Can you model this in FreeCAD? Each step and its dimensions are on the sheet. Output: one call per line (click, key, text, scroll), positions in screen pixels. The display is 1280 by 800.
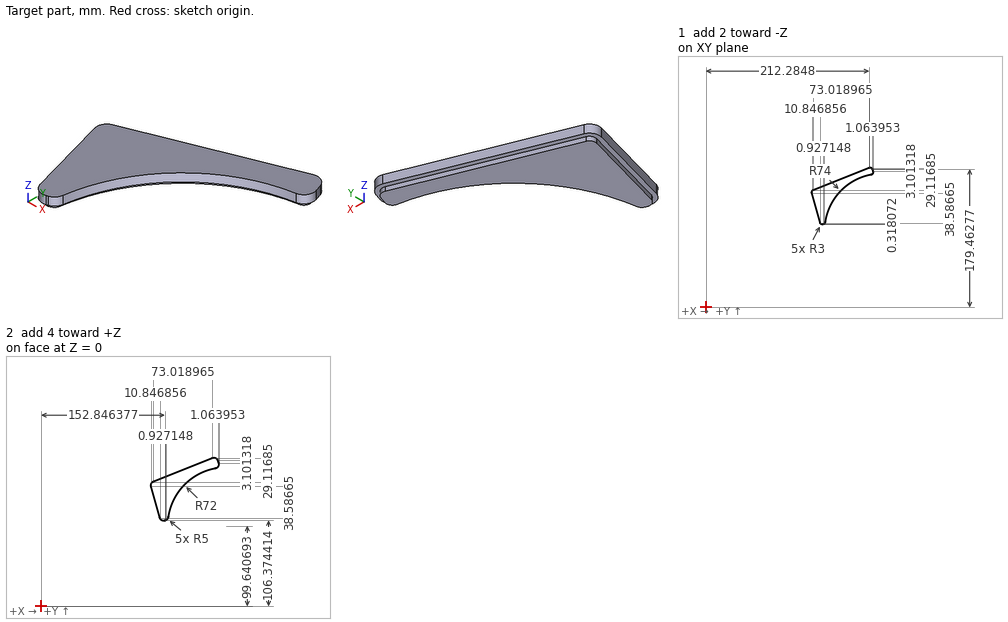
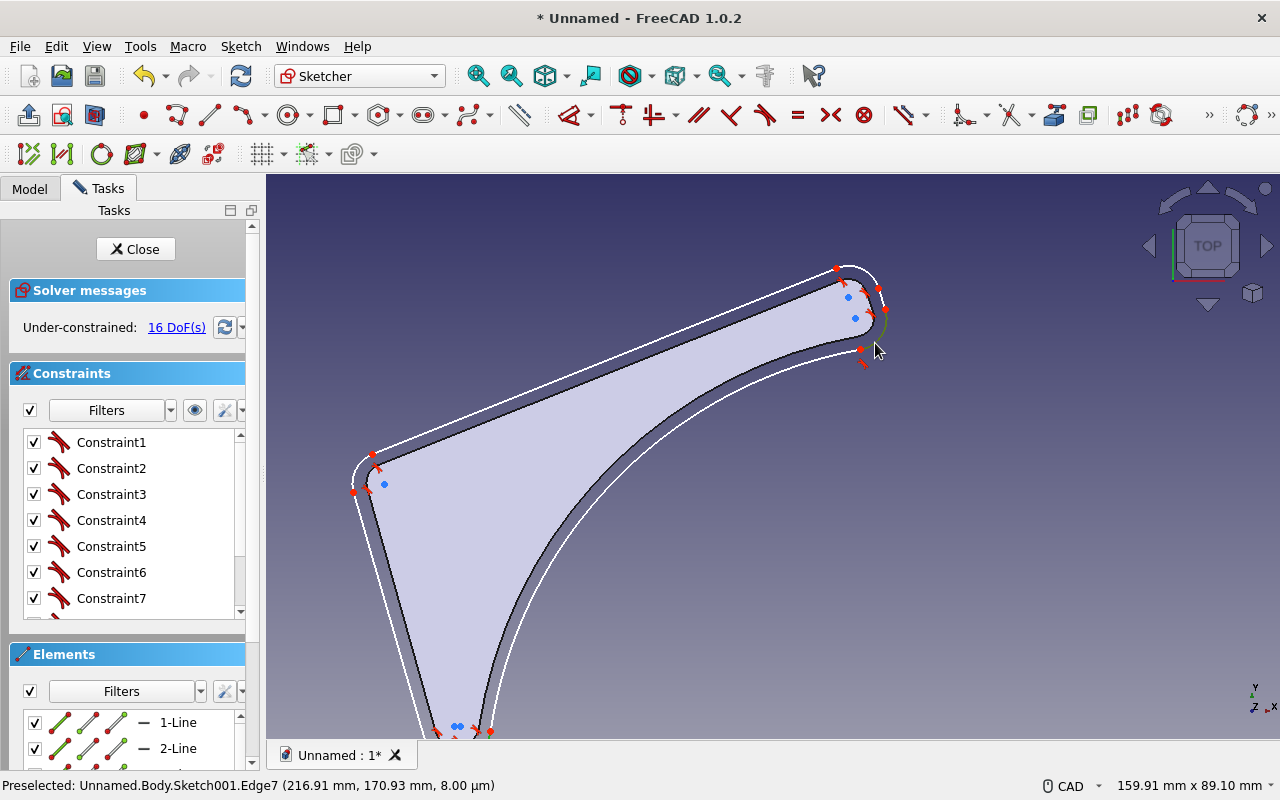
click(871, 275)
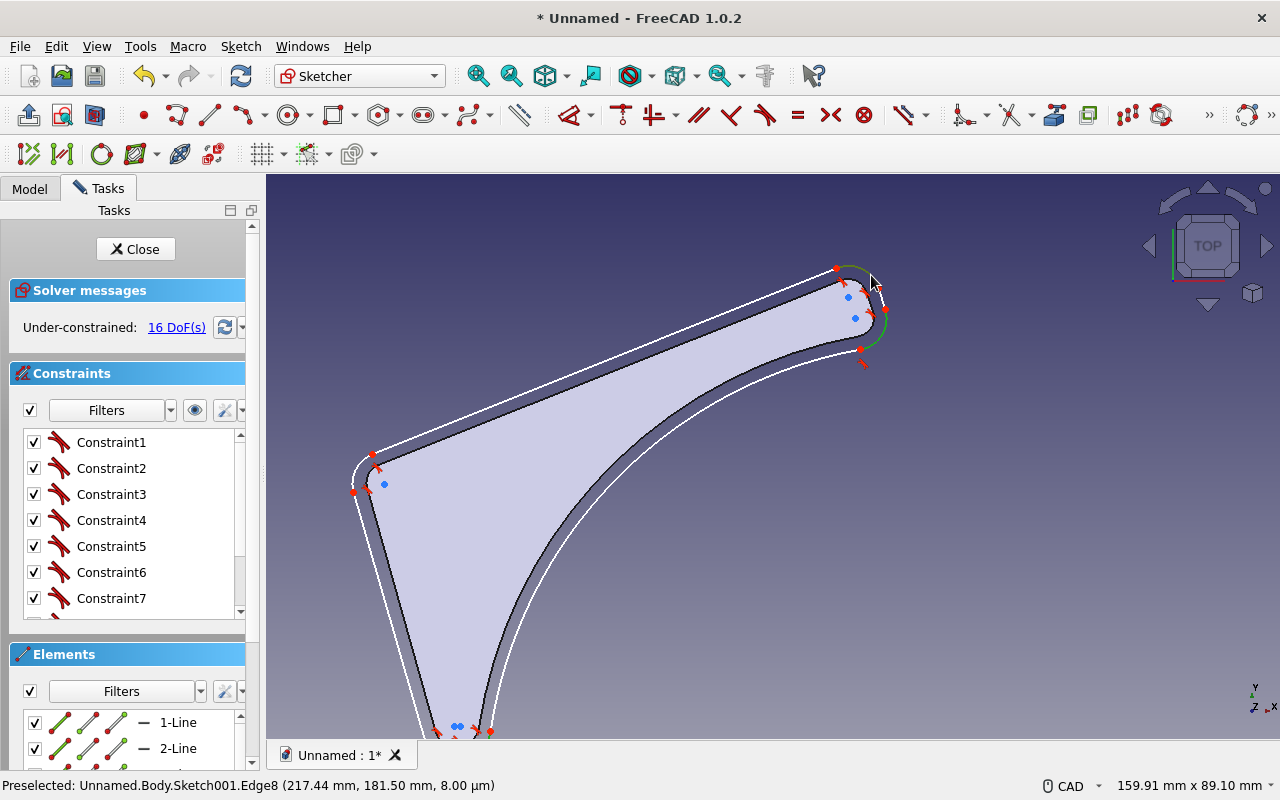
click(361, 462)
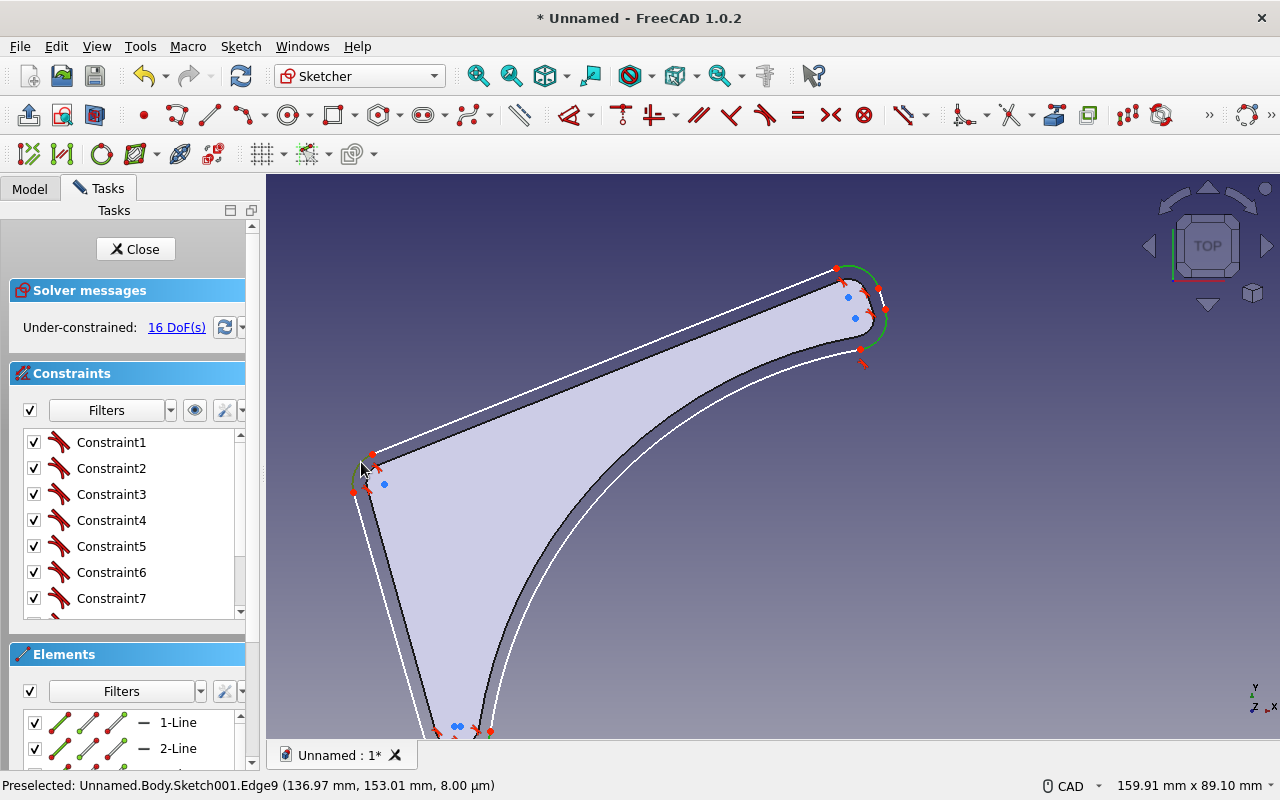
scroll(876, 342, down, 2)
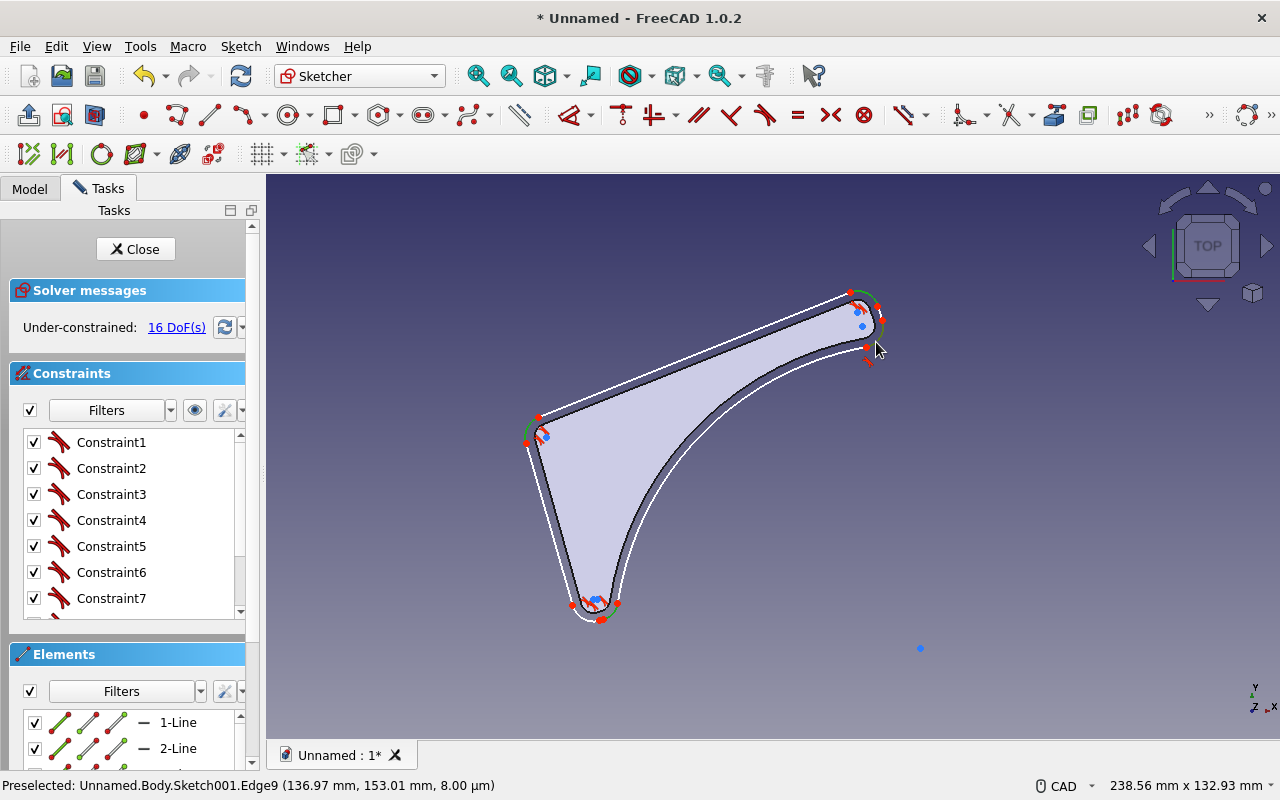
scroll(578, 615, up, 2)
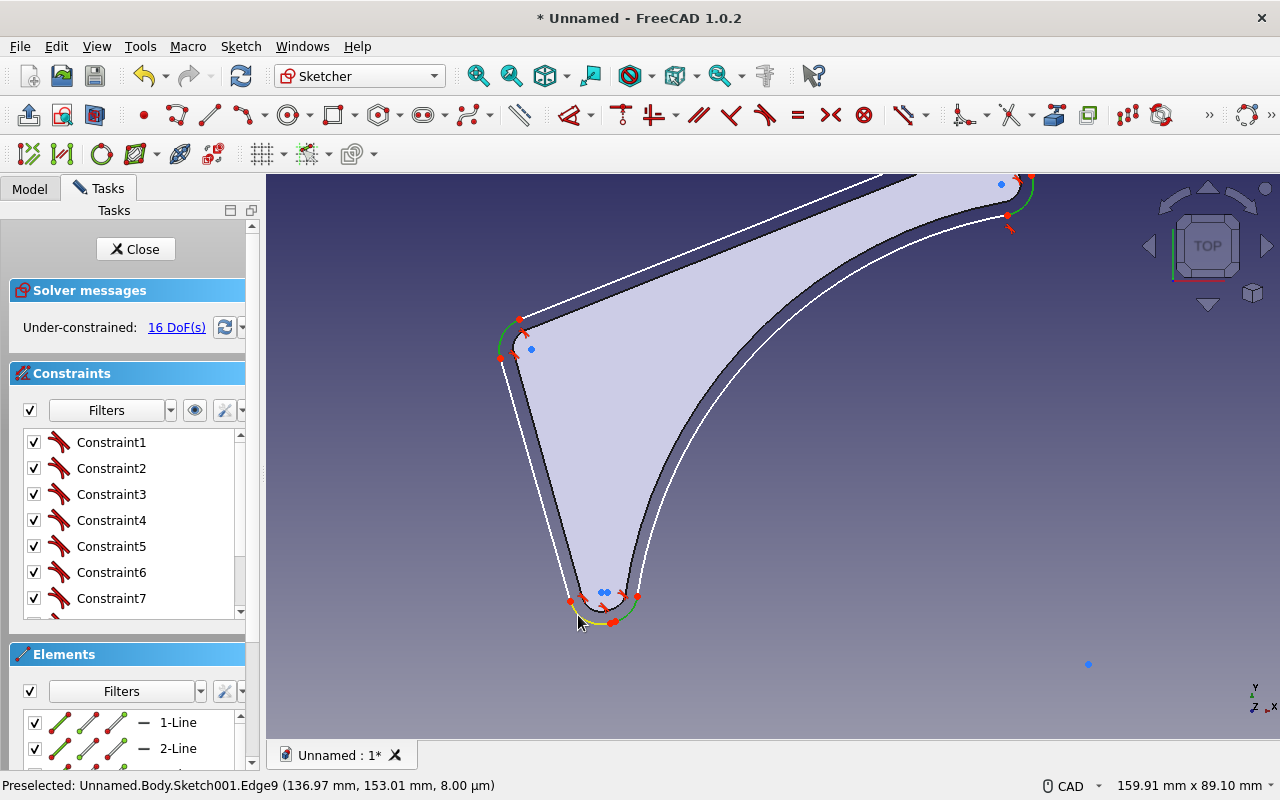
click(578, 614)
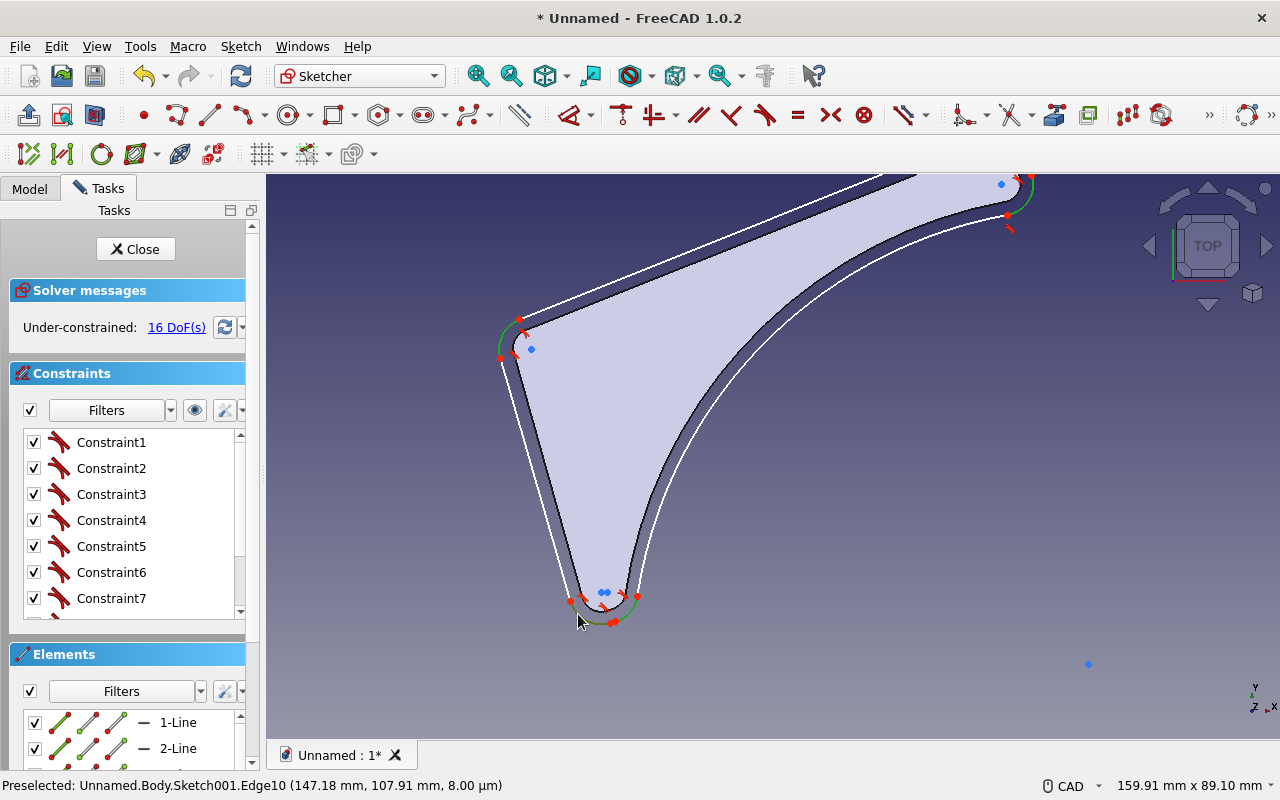
click(798, 116)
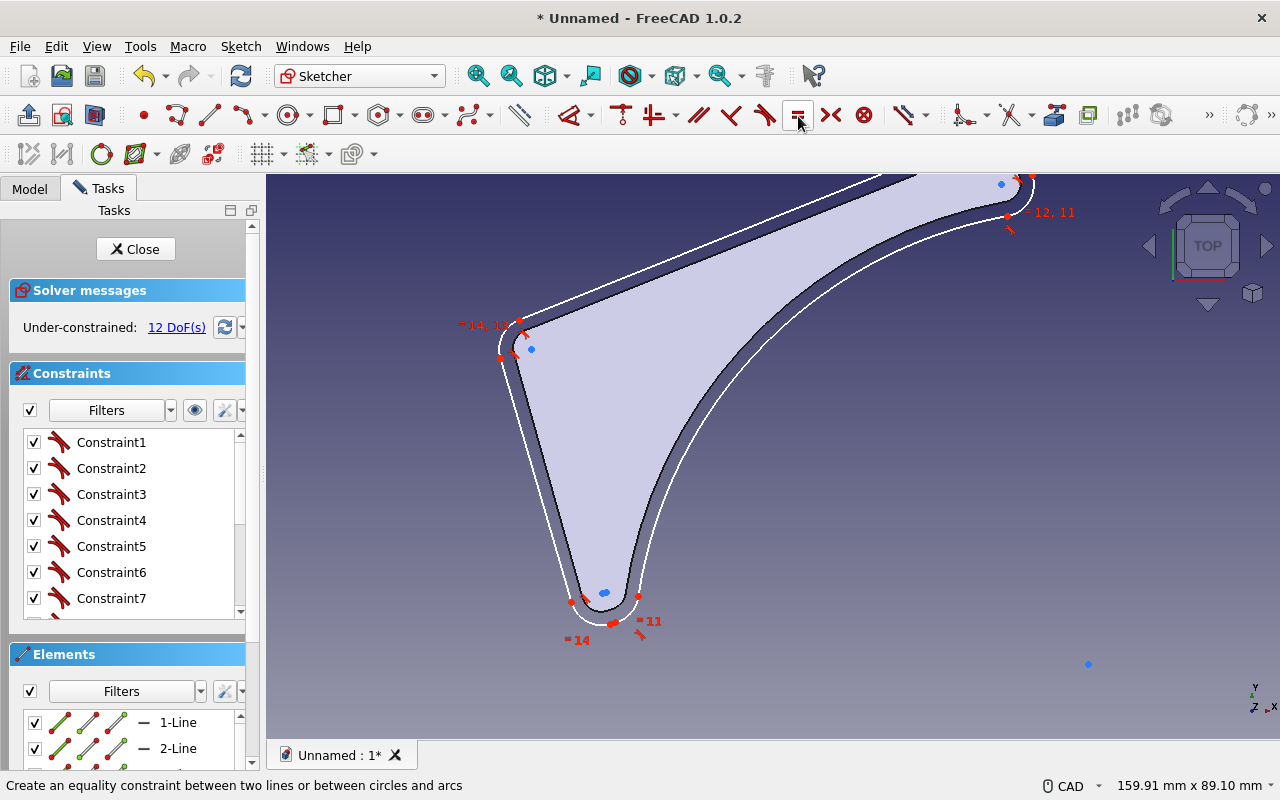
click(568, 116)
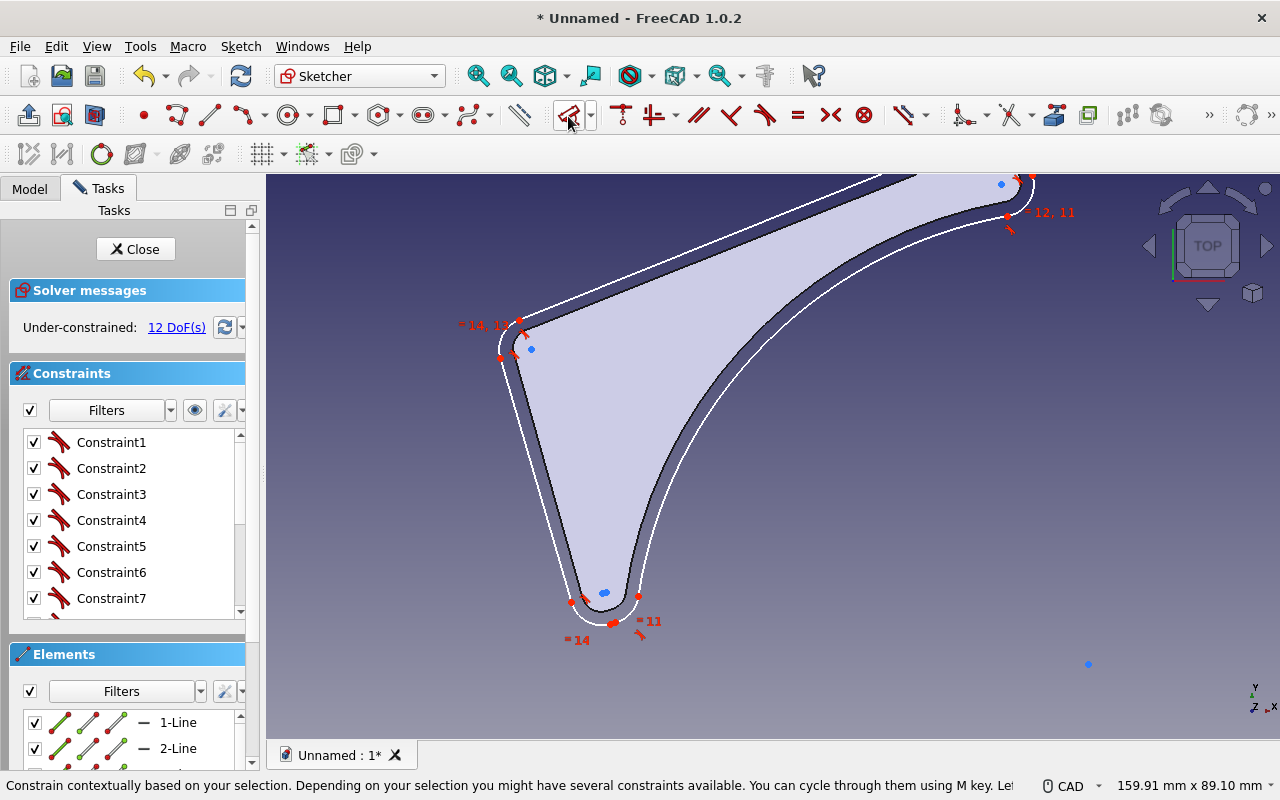
scroll(625, 618, up, 2)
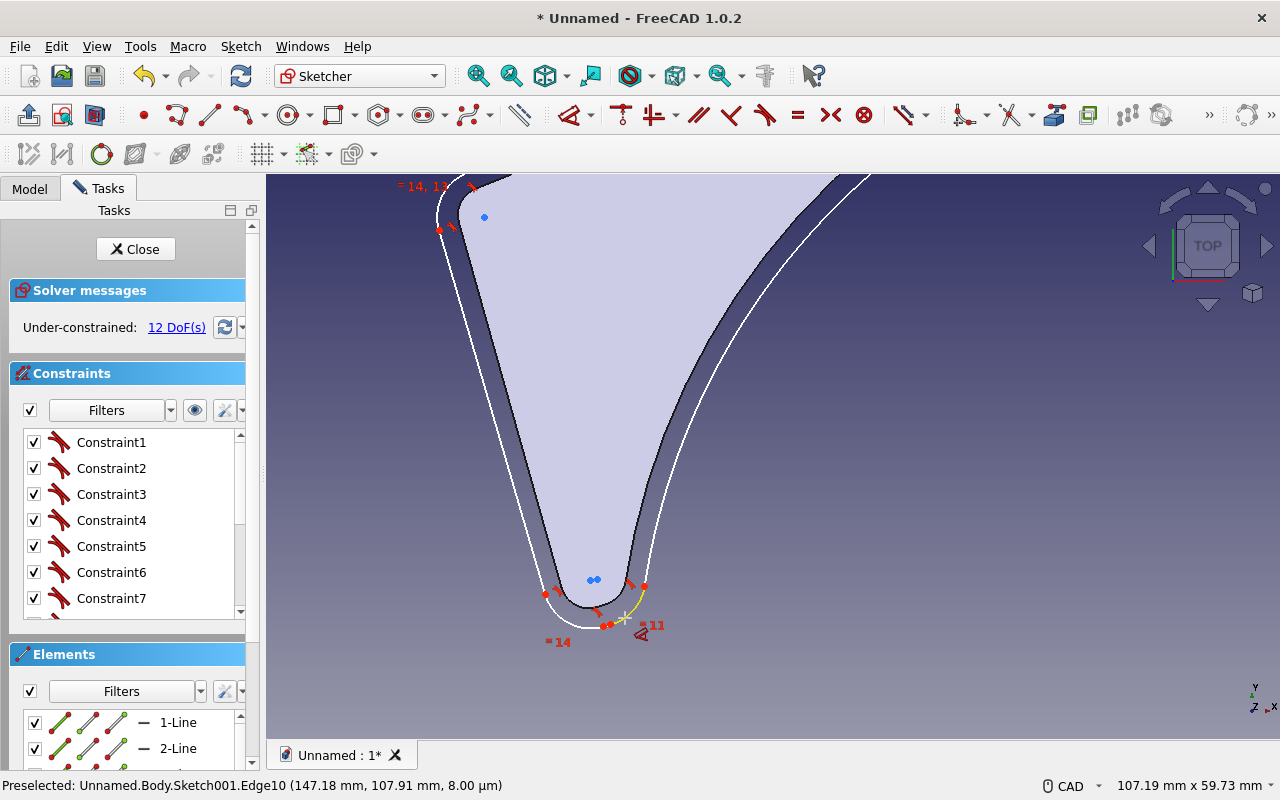
click(625, 618)
click(643, 644)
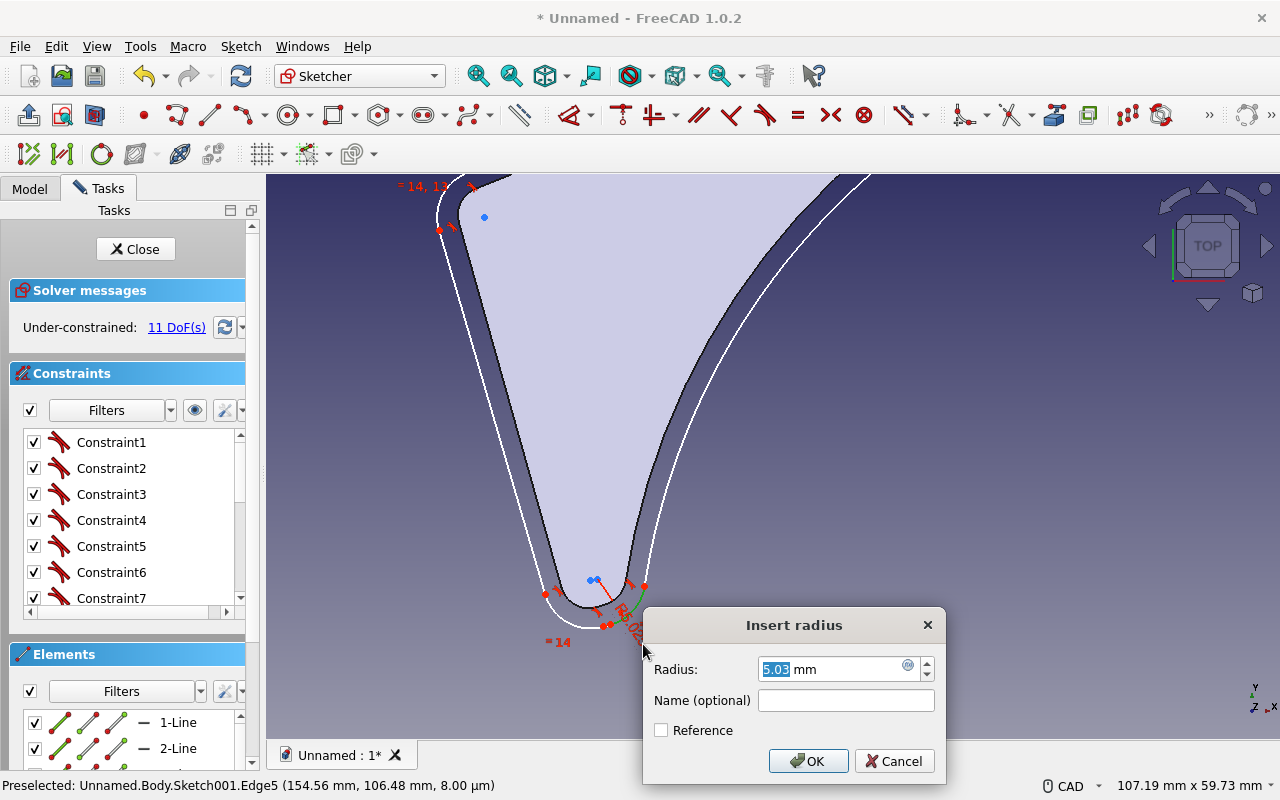
text(5)
key(Return)